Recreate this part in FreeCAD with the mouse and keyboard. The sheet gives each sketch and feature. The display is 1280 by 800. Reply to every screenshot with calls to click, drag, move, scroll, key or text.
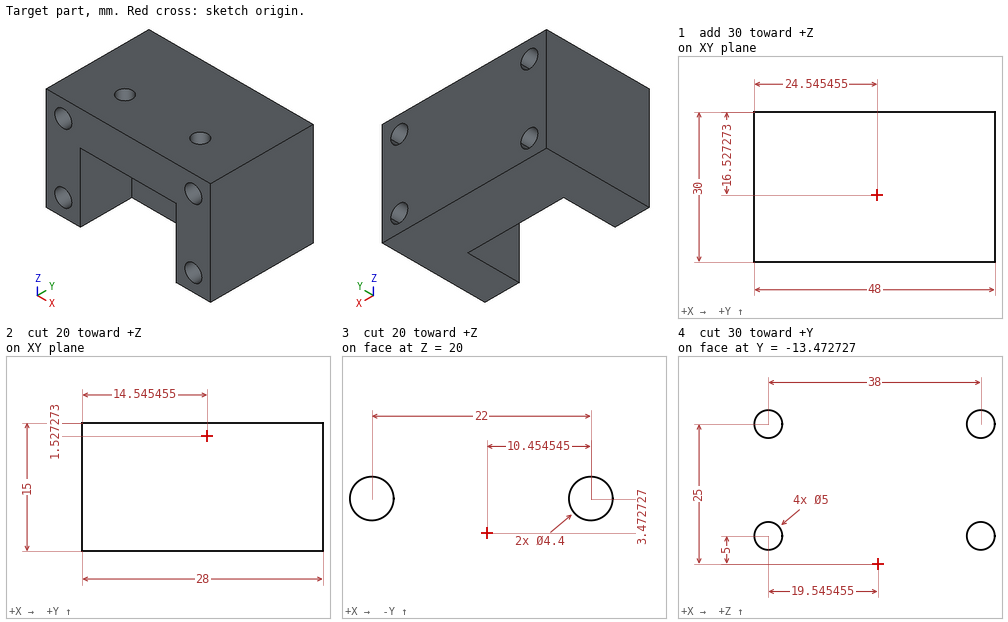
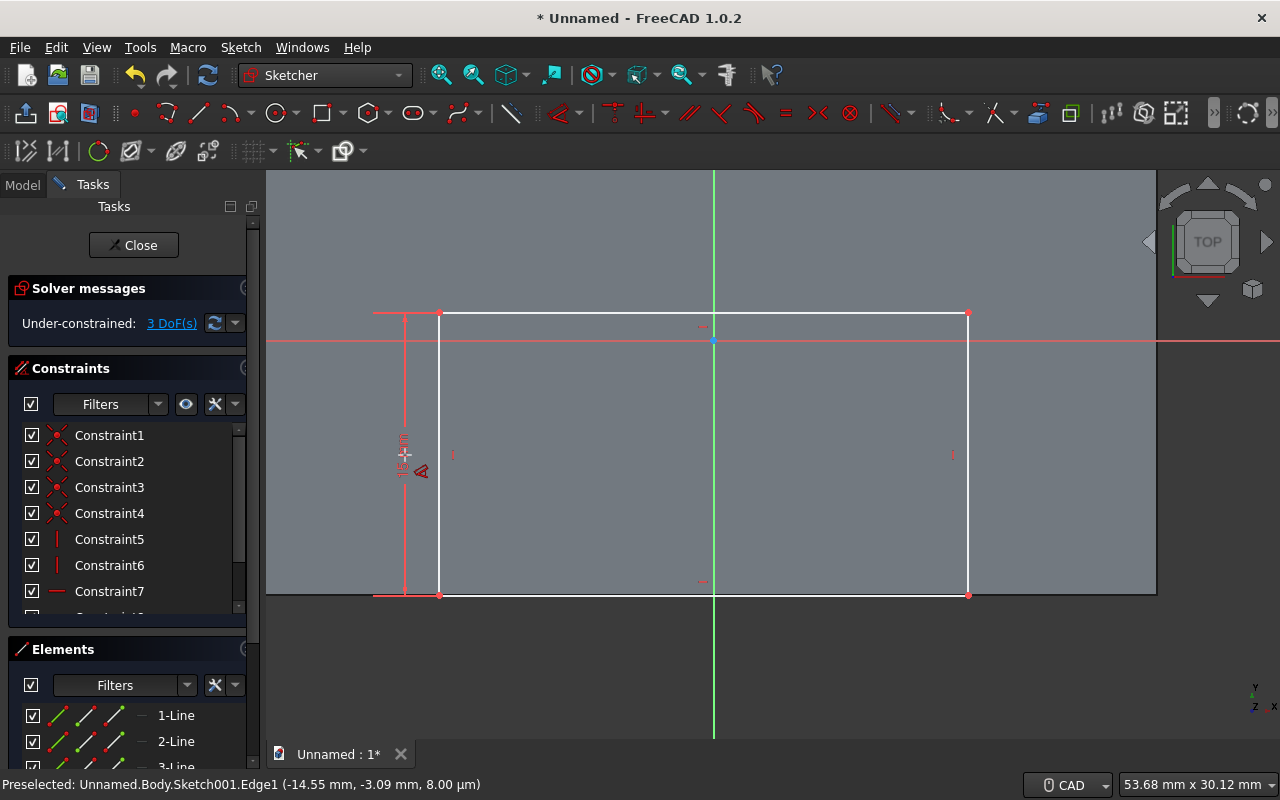
click(598, 596)
click(582, 630)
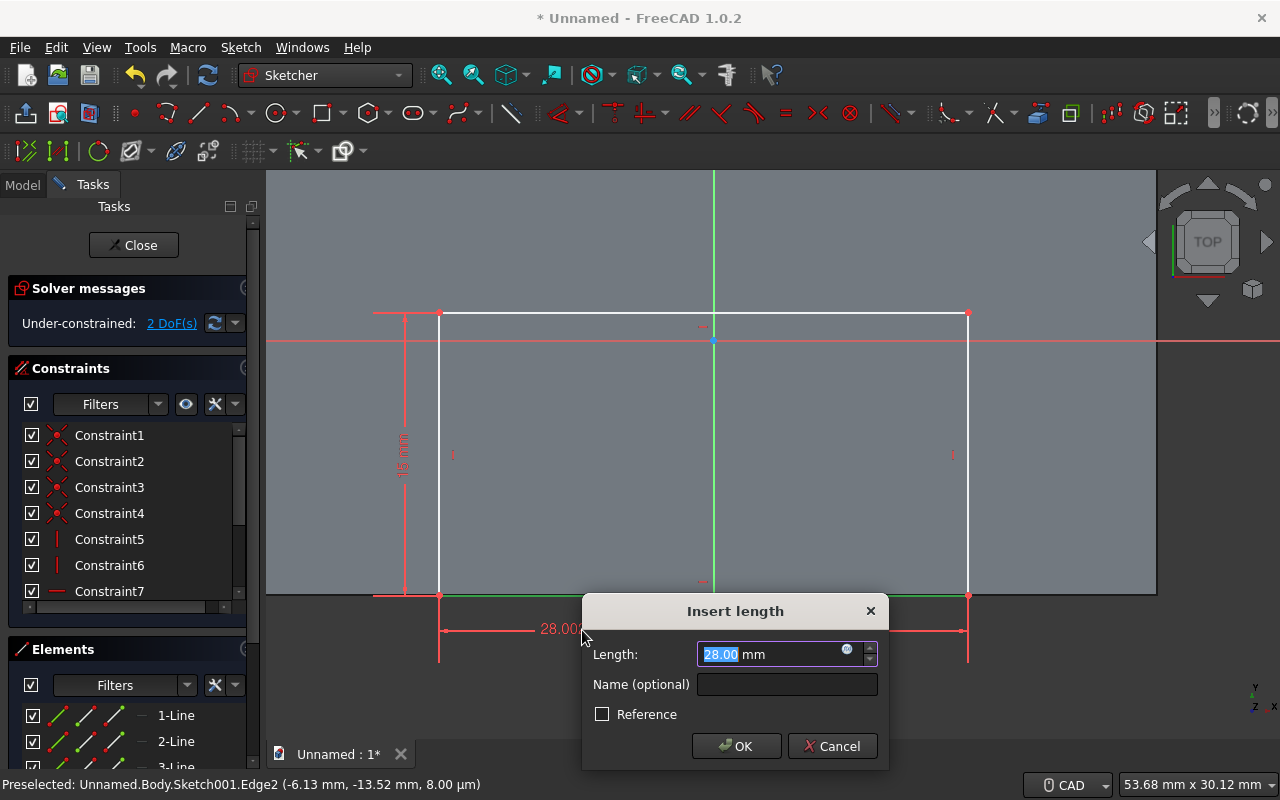
text(28)
key(Return)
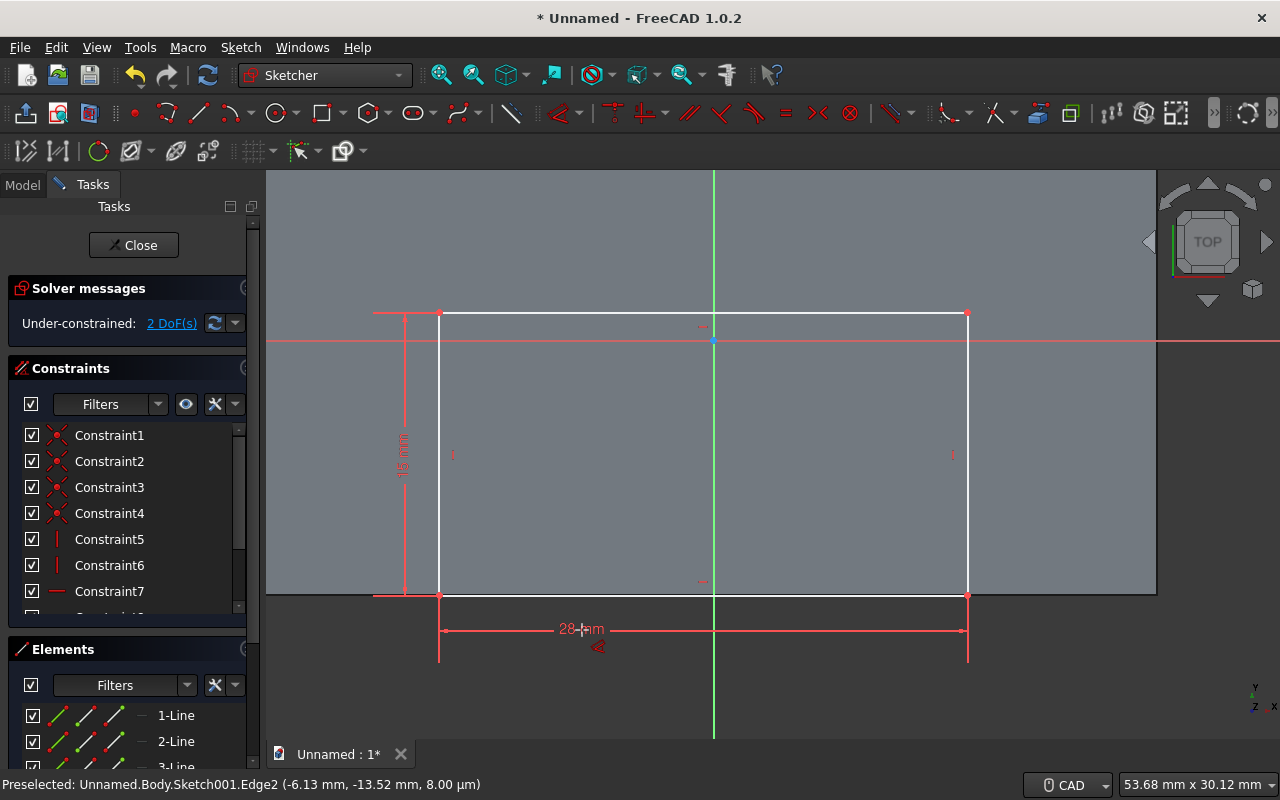
scroll(439, 313, up, 2)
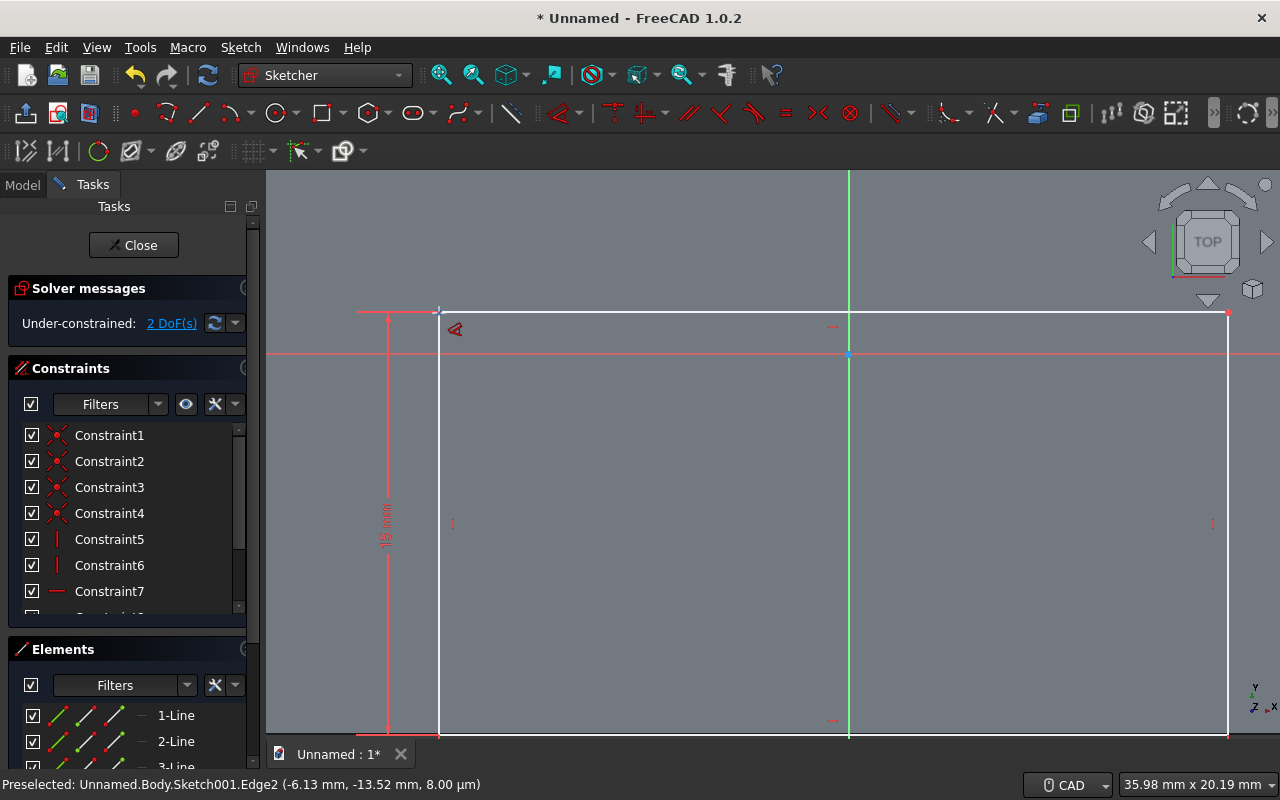
click(439, 312)
click(405, 333)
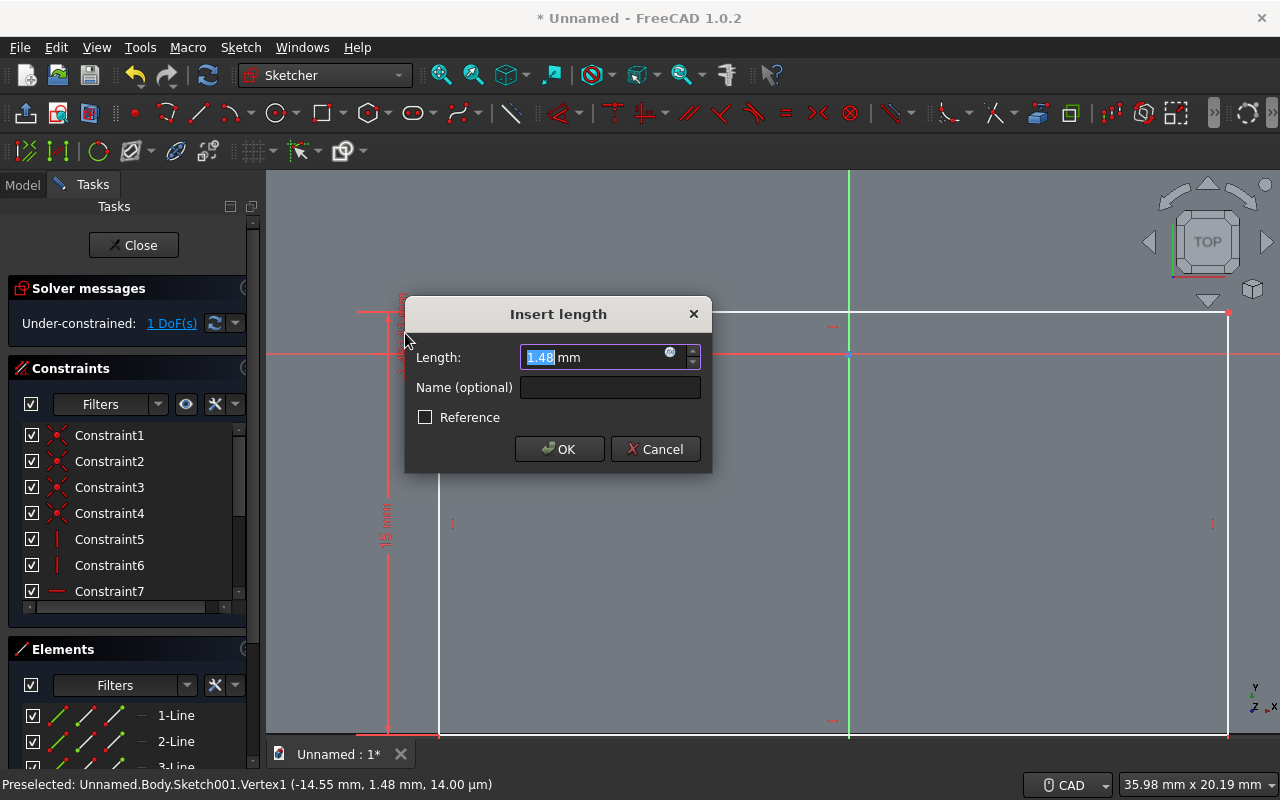
text(1.527273)
key(Return)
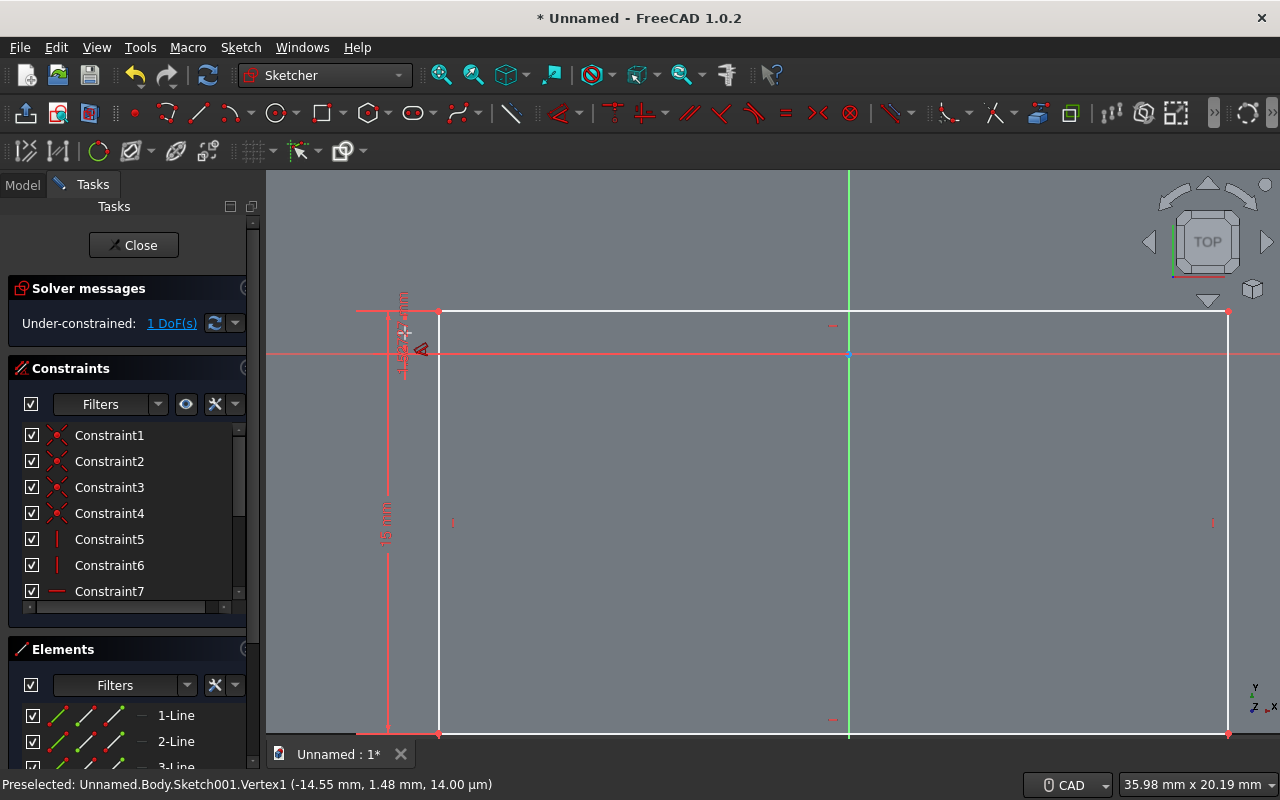
click(439, 311)
click(644, 277)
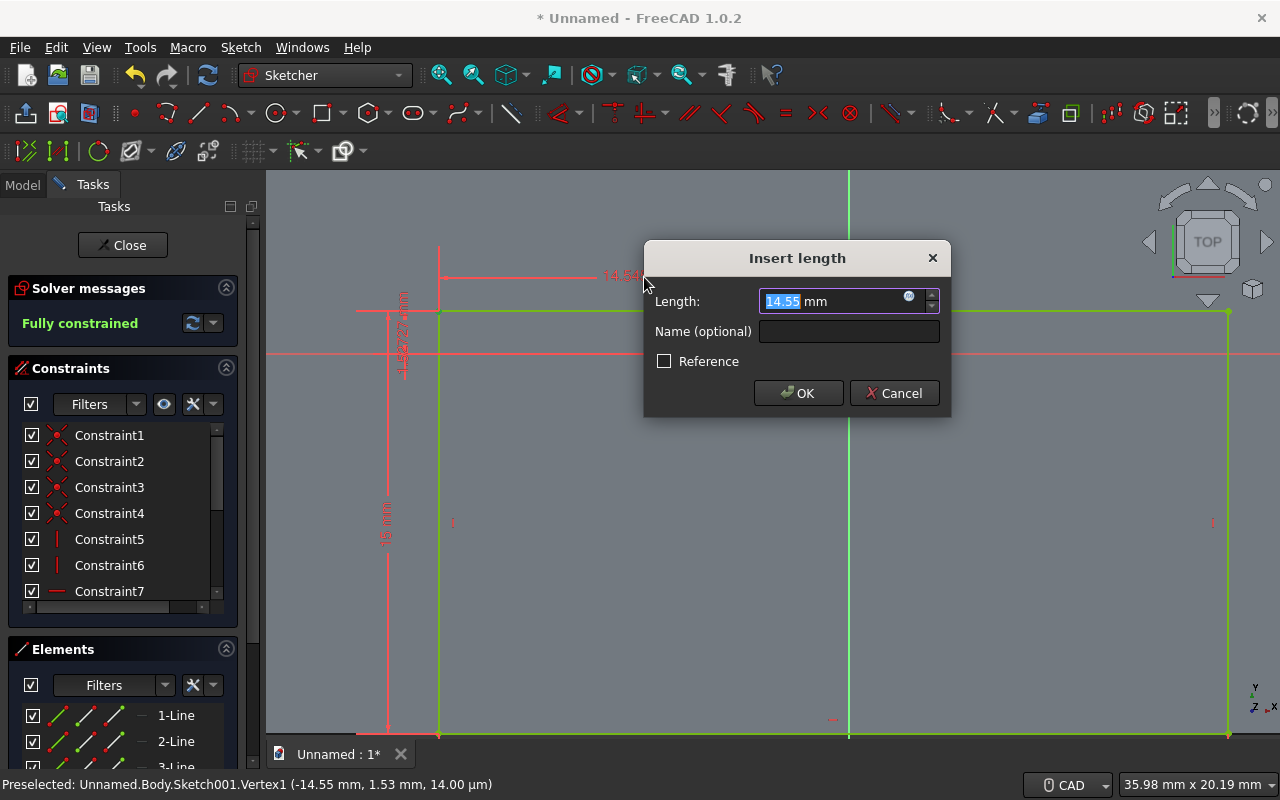
text(14.545455)
key(Return)
key(Escape)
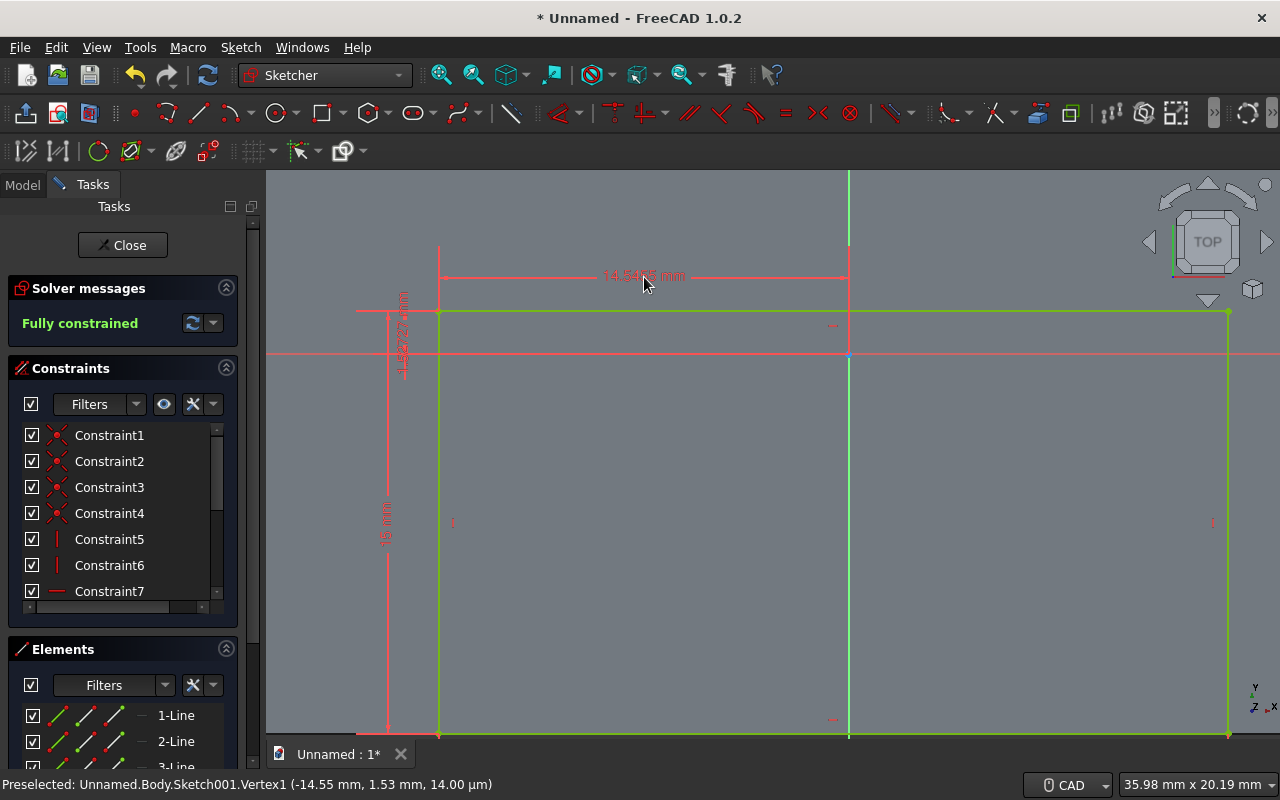
click(123, 245)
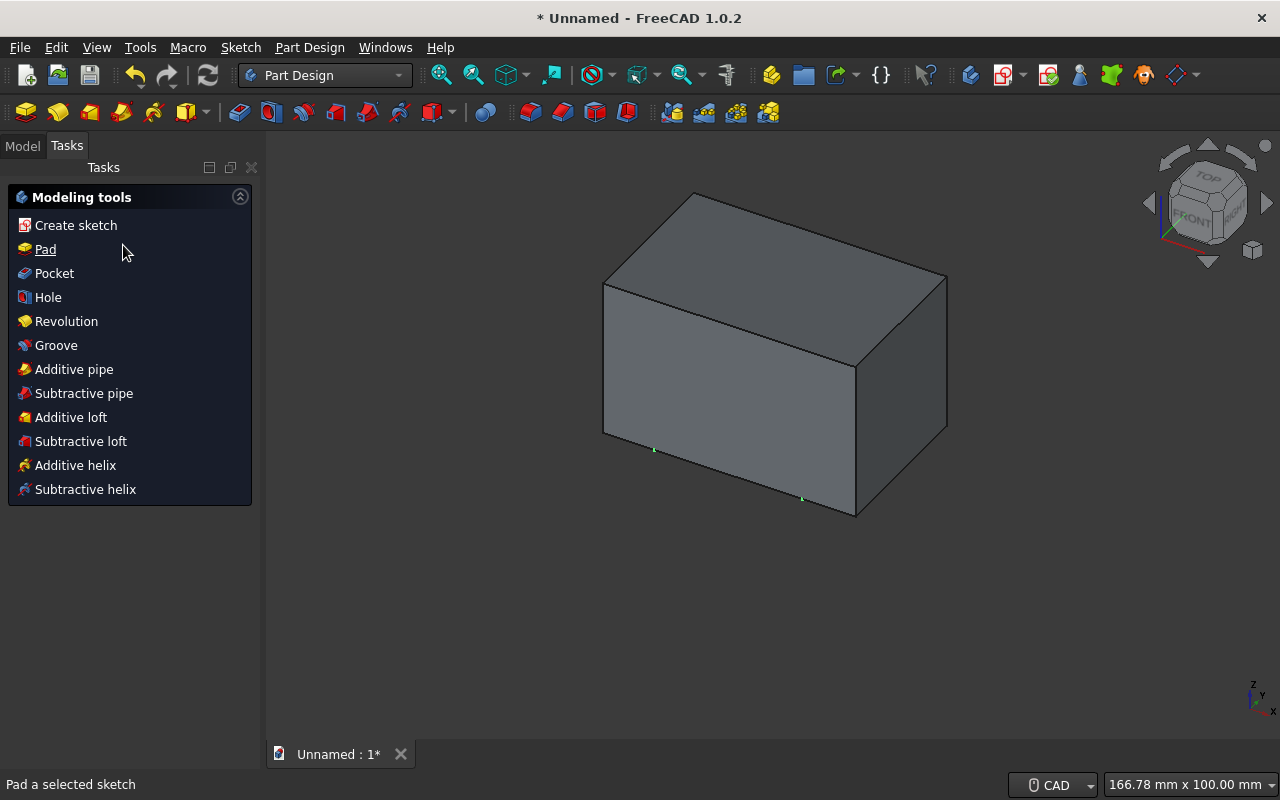
click(240, 112)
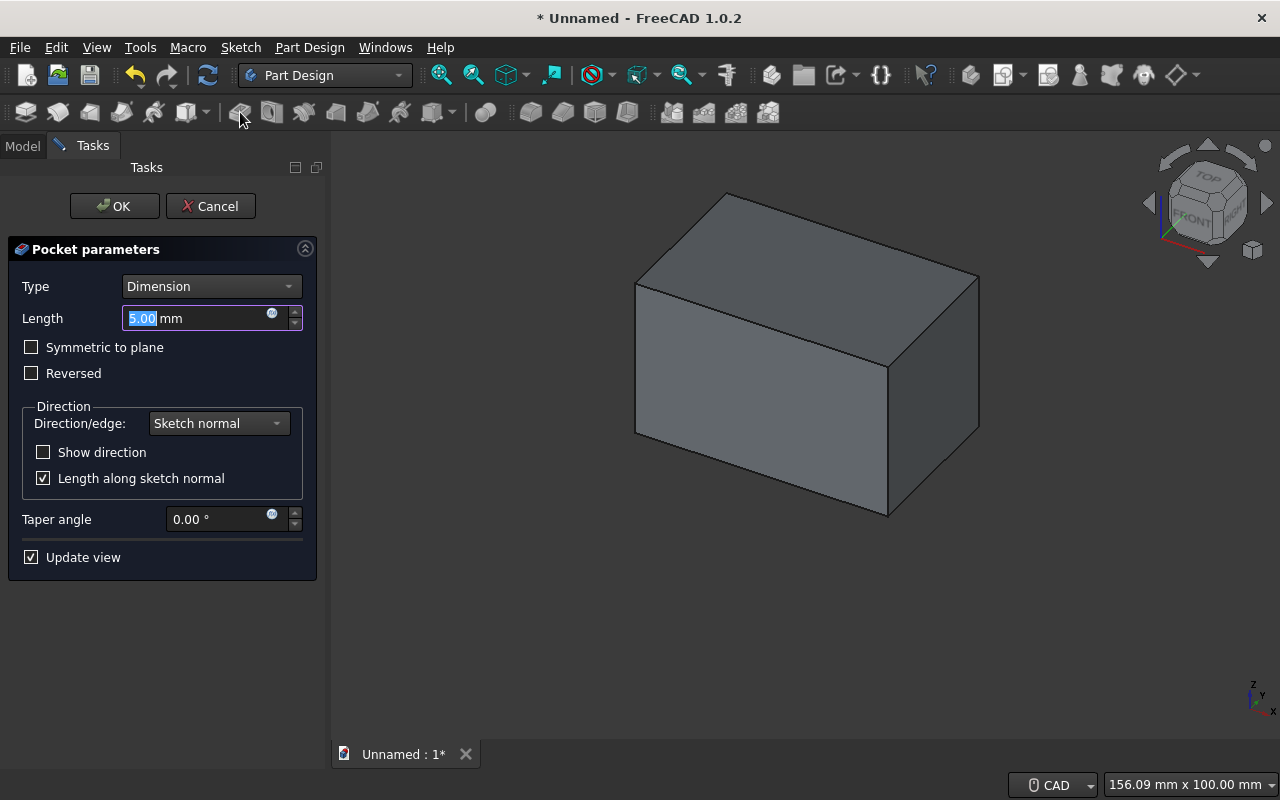
text(20)
key(Tab)